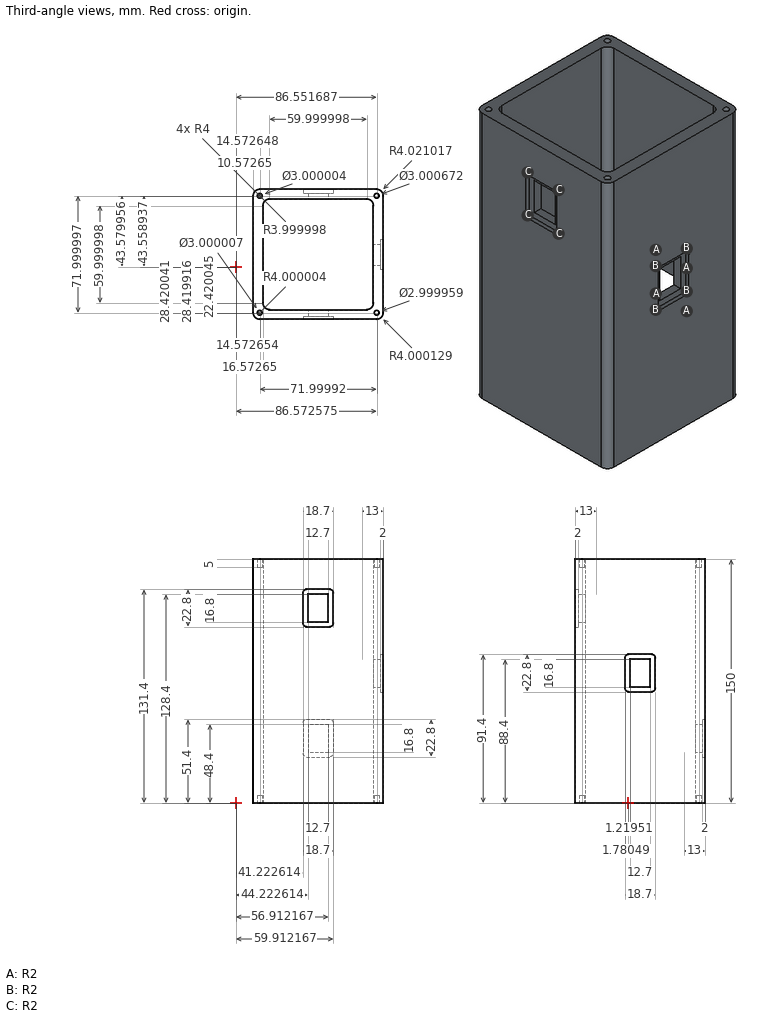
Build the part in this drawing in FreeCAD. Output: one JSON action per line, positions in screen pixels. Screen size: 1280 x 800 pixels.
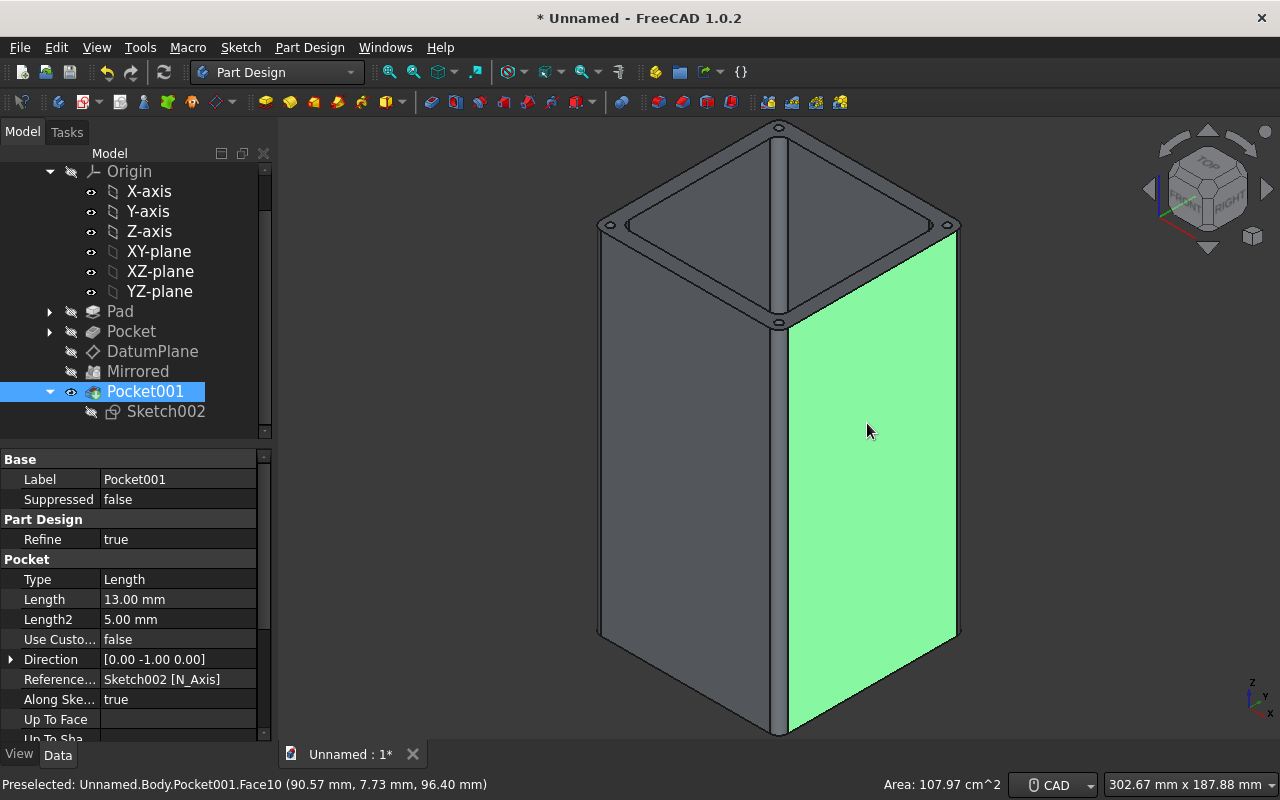
{"action": "left_click", "coordinate": [84, 102]}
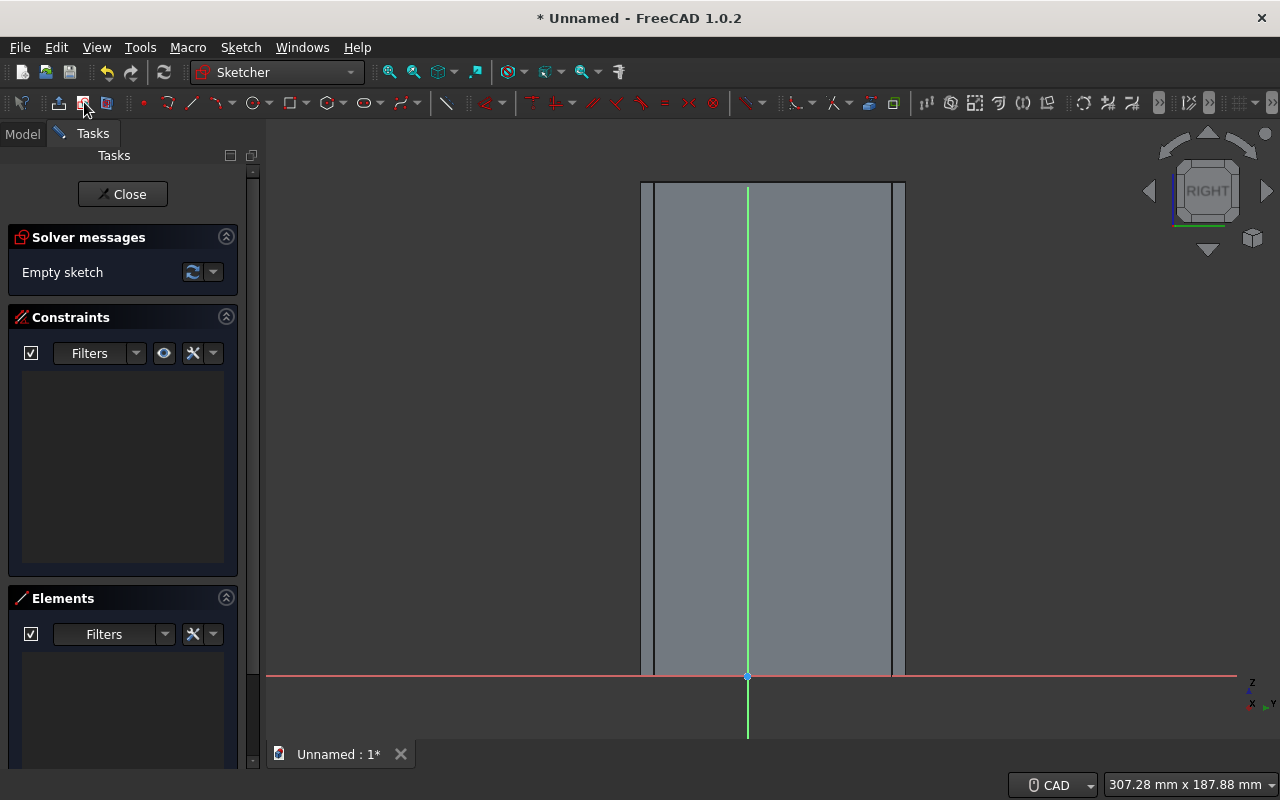
{"action": "scroll", "coordinate": [784, 410], "scroll_direction": "up", "scroll_amount": 10}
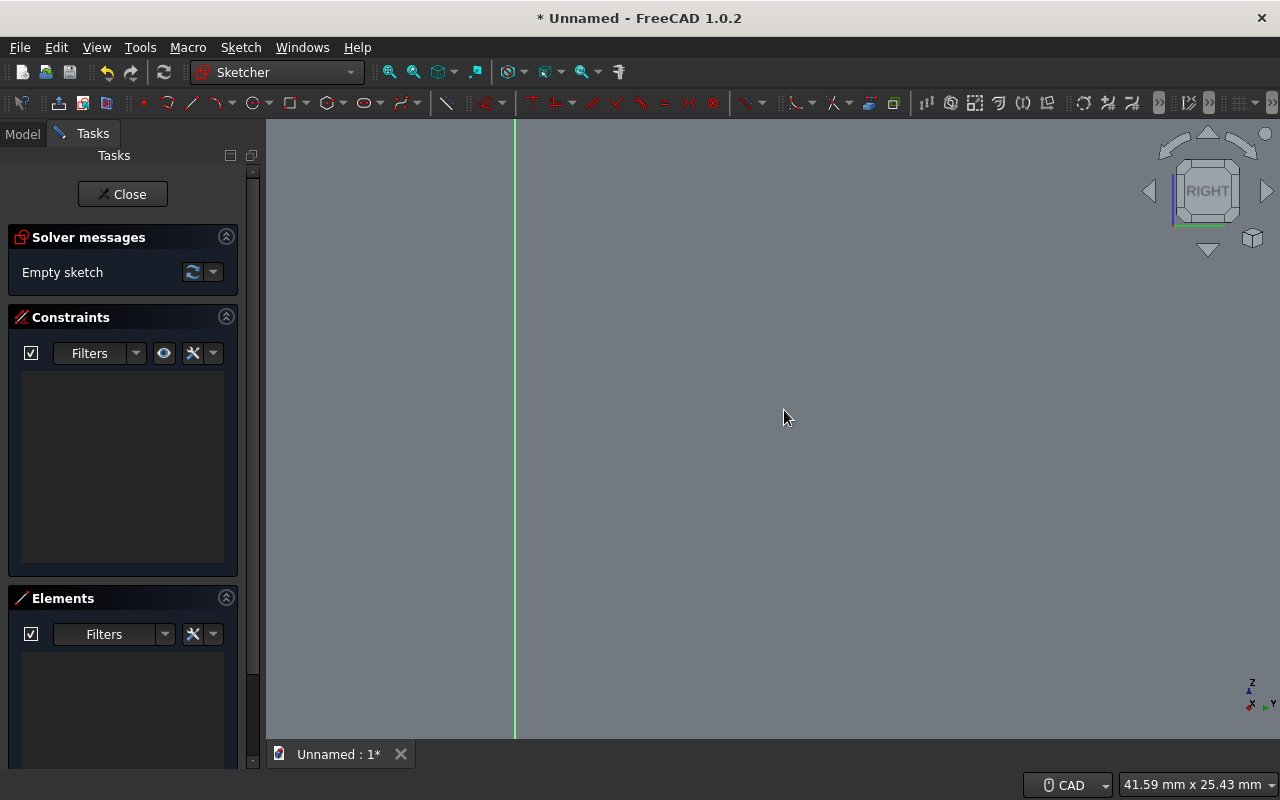
{"action": "left_click", "coordinate": [290, 104]}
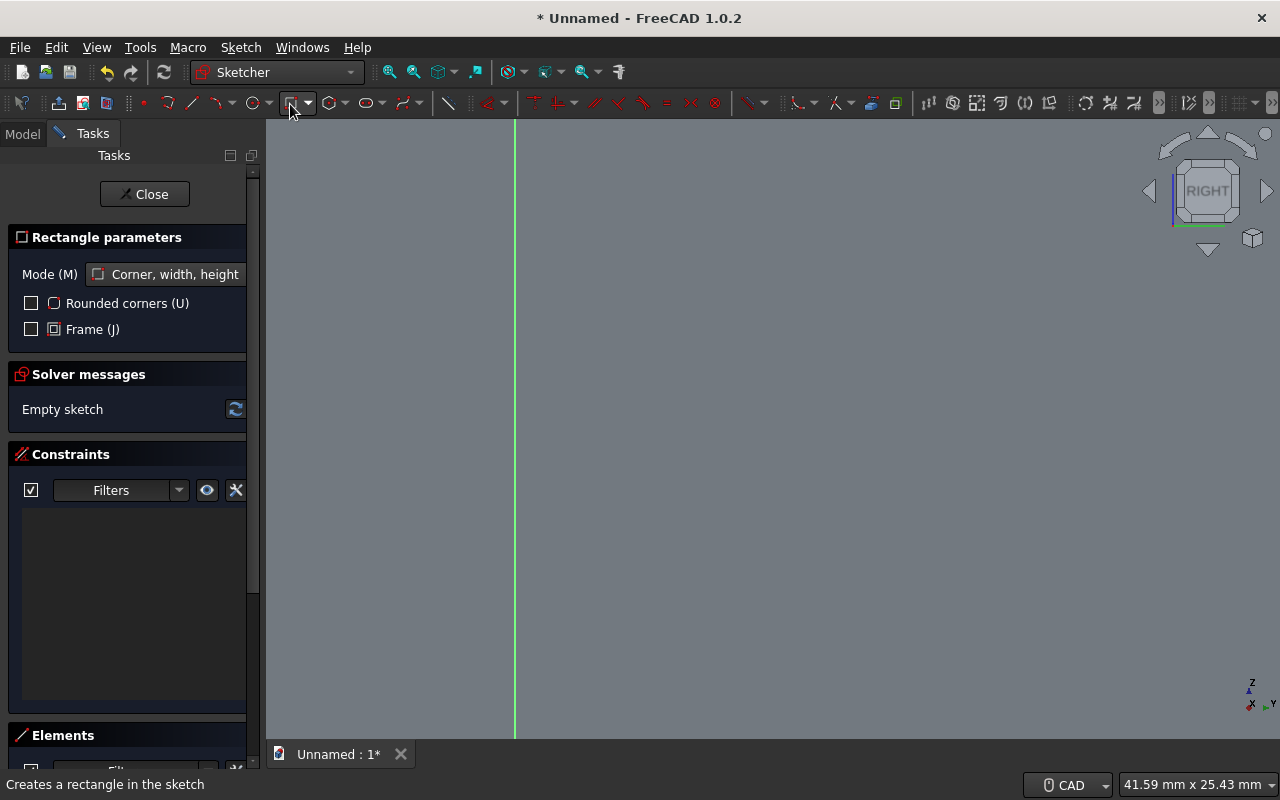
{"action": "left_click", "coordinate": [544, 221]}
{"action": "left_click", "coordinate": [854, 630]}
{"action": "key", "text": "Escape"}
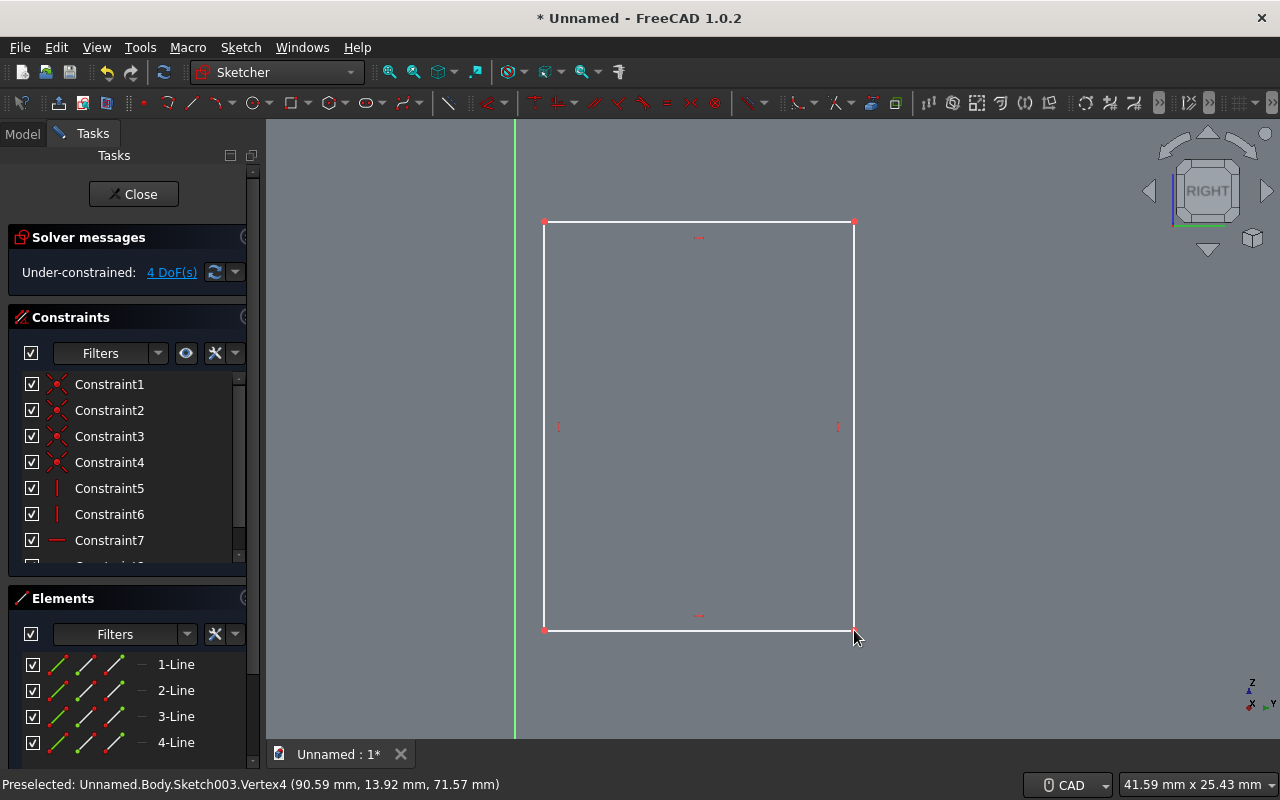
{"action": "left_click", "coordinate": [488, 104]}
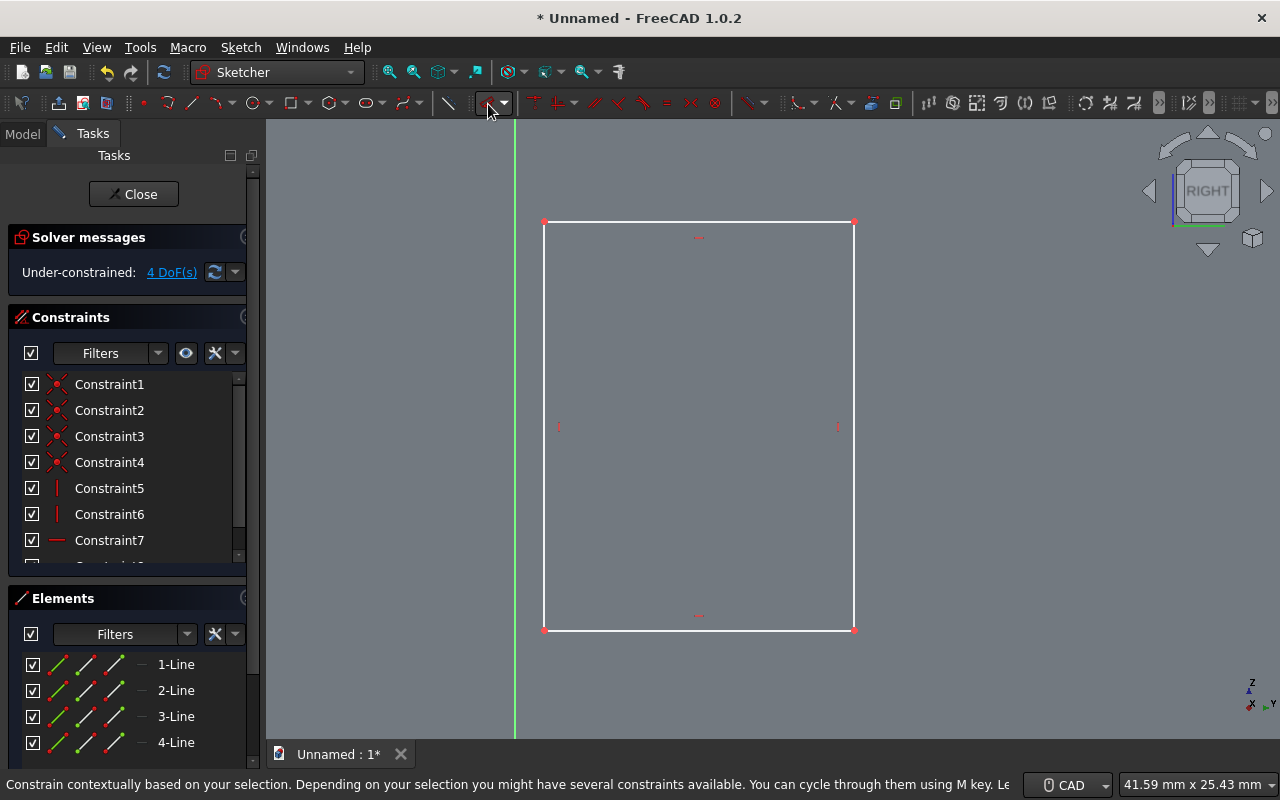
{"action": "left_click", "coordinate": [544, 345]}
{"action": "left_click", "coordinate": [578, 427]}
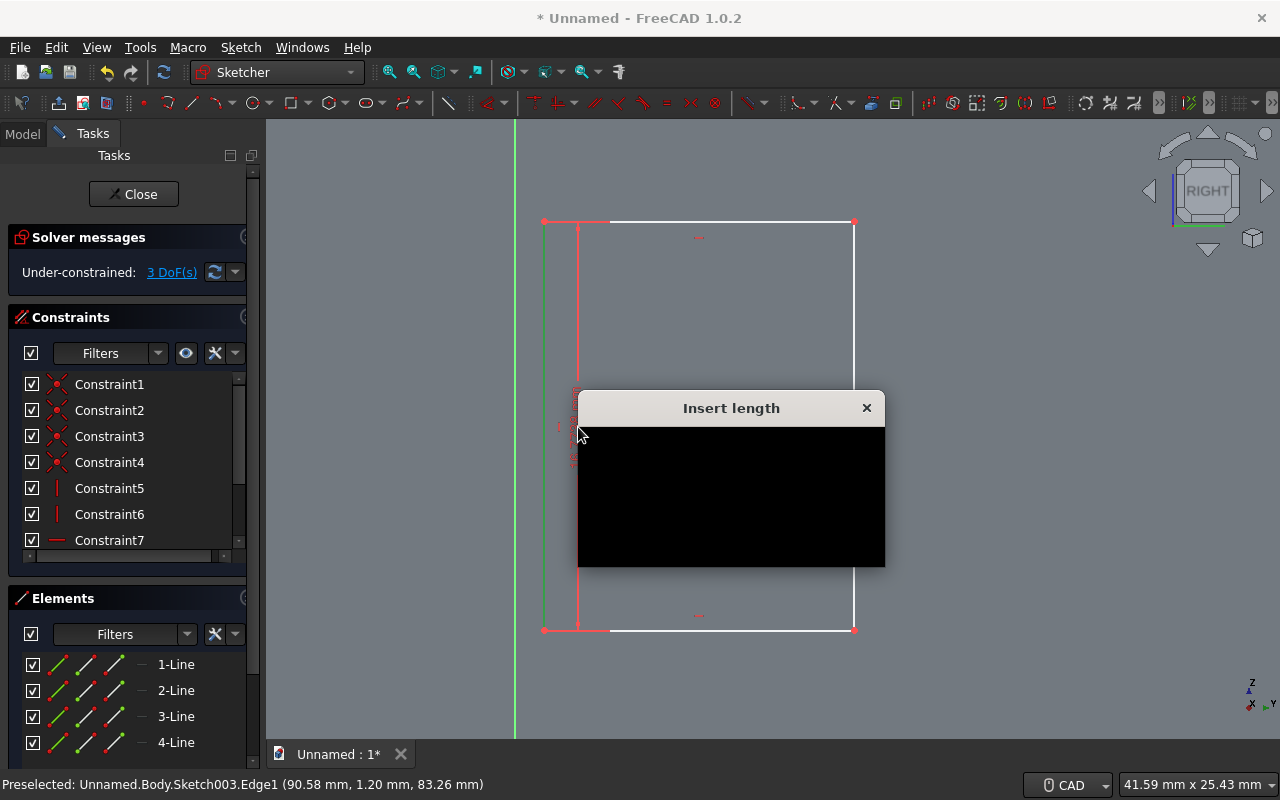
{"action": "type", "text": "16.8"}
{"action": "key", "text": "Return"}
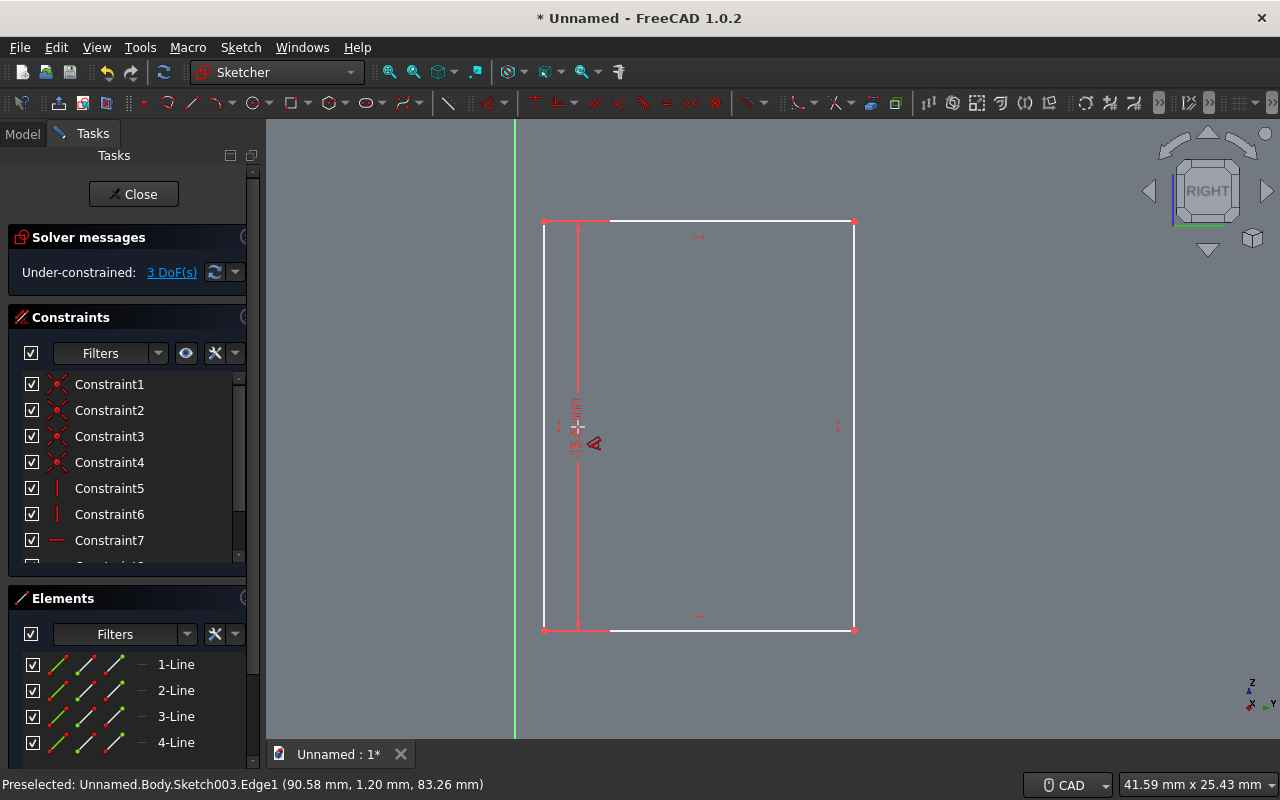
{"action": "left_click", "coordinate": [637, 631]}
{"action": "left_click", "coordinate": [699, 665]}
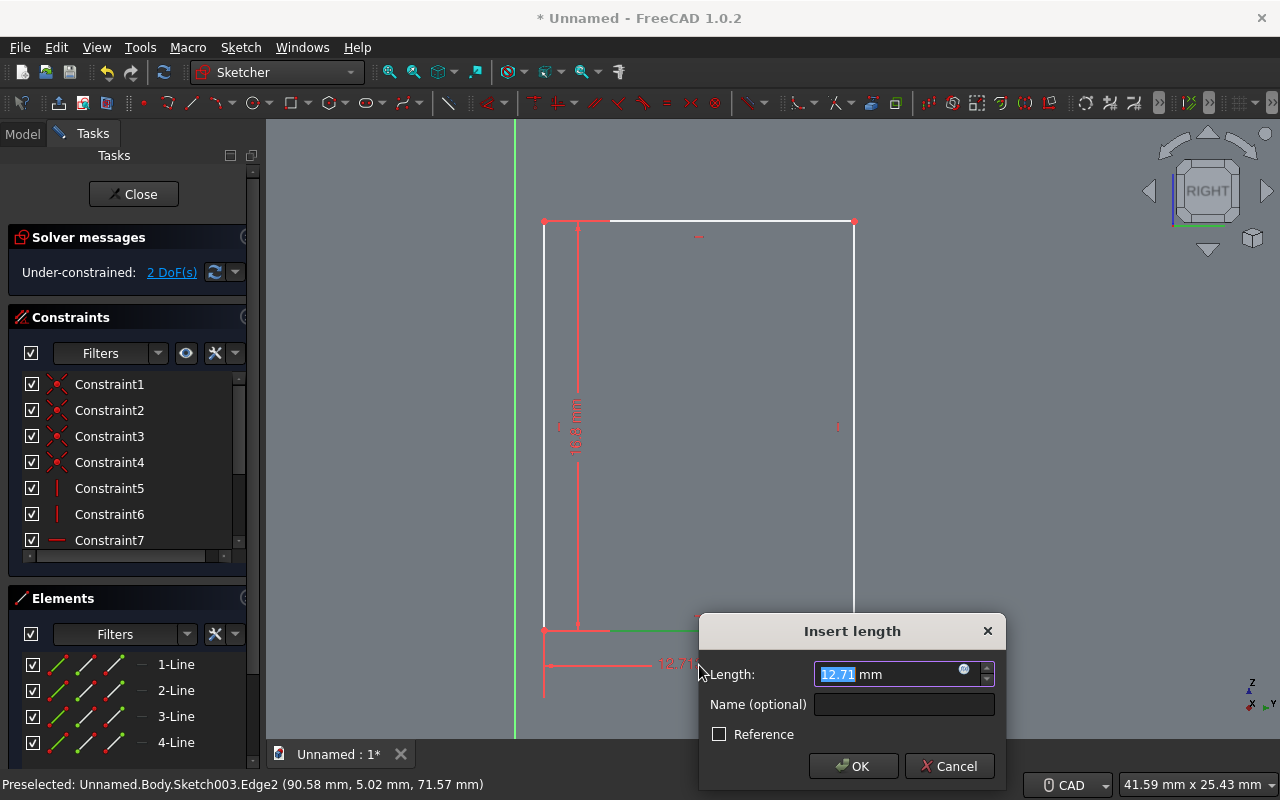
{"action": "type", "text": "12.7"}
{"action": "key", "text": "Return"}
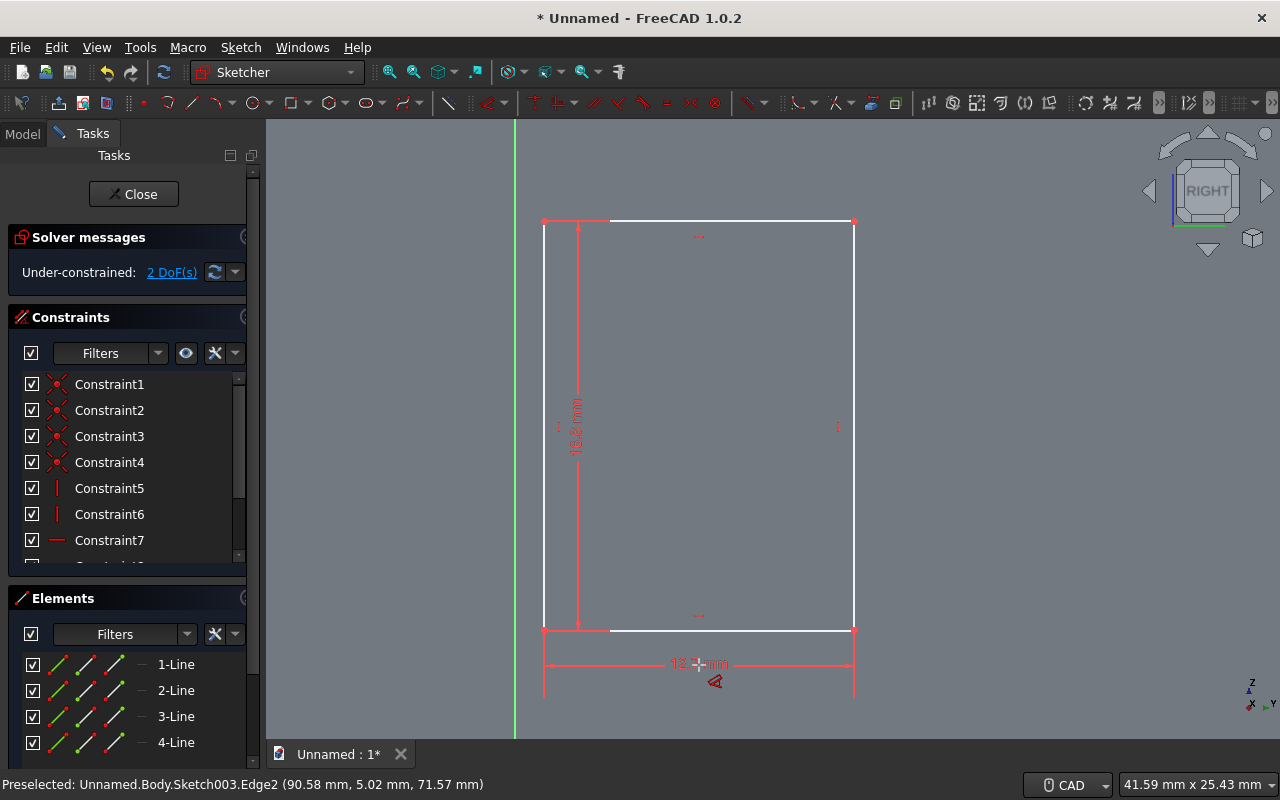
{"action": "left_click", "coordinate": [544, 221]}
{"action": "left_click", "coordinate": [481, 466]}